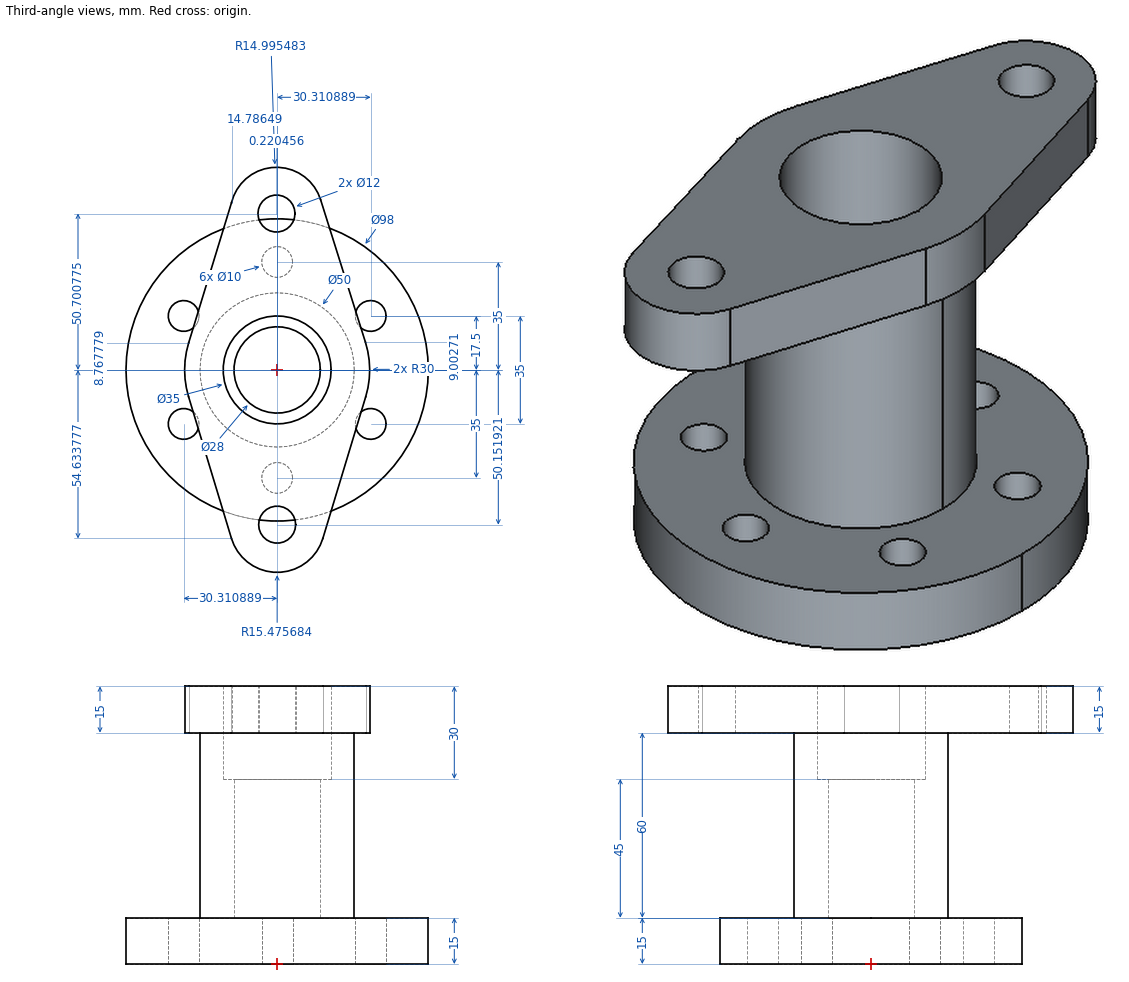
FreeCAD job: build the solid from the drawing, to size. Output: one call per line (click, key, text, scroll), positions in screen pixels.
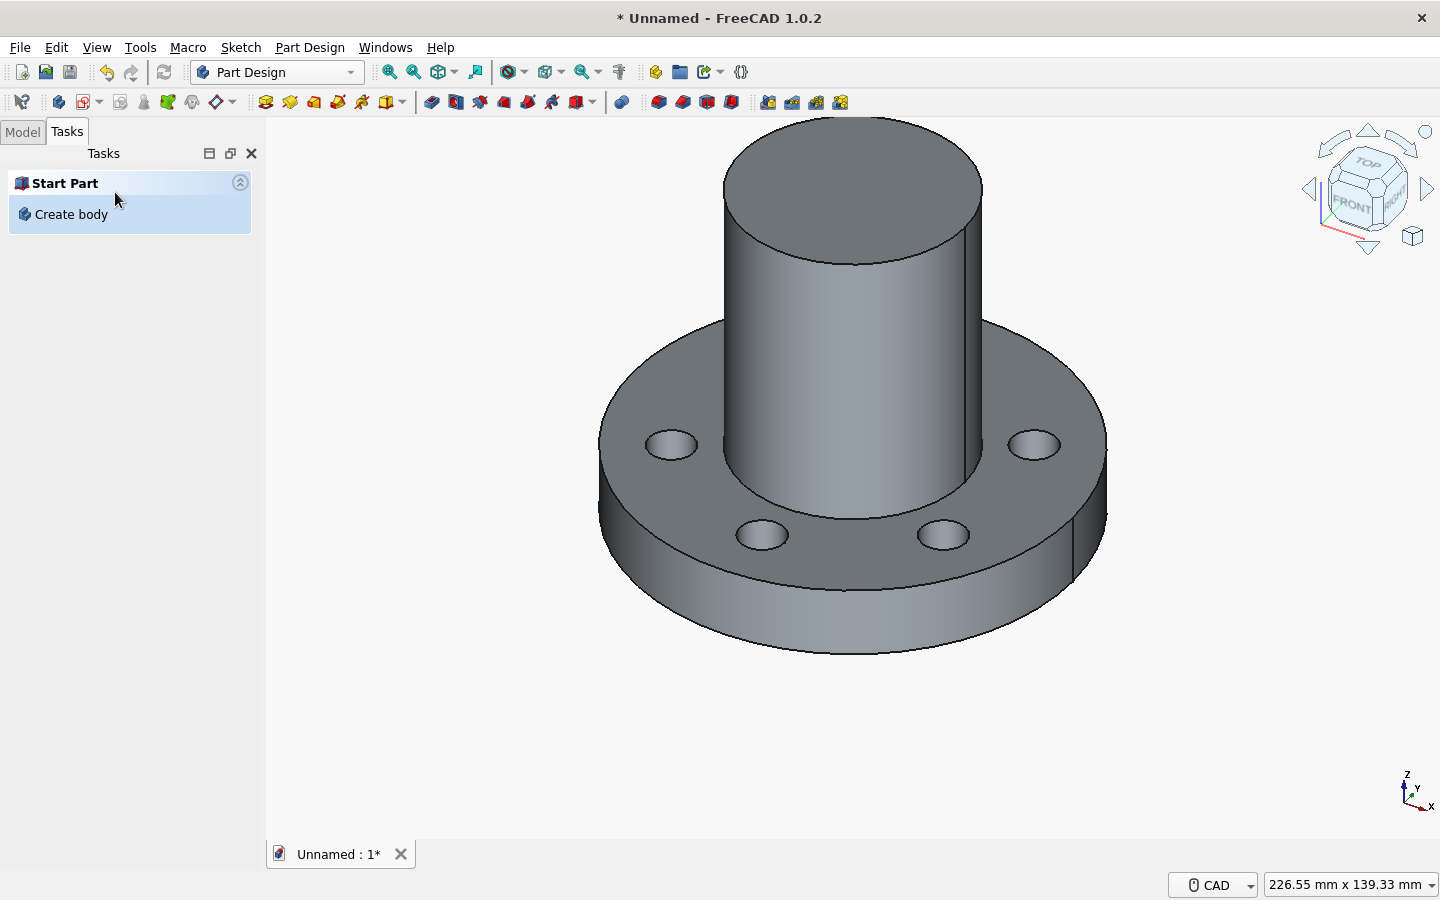
click(390, 72)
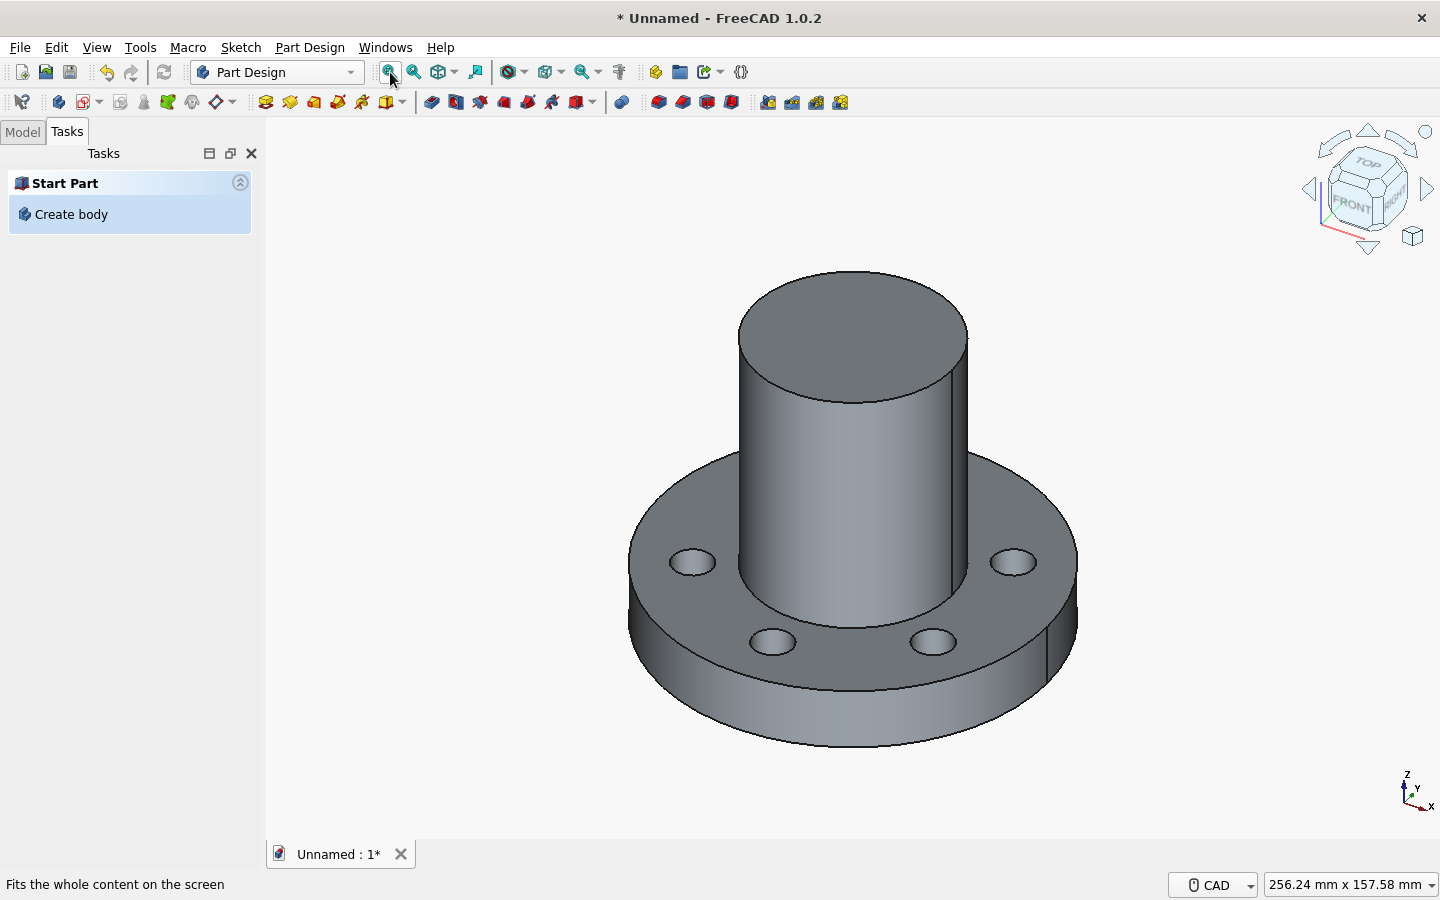
click(853, 336)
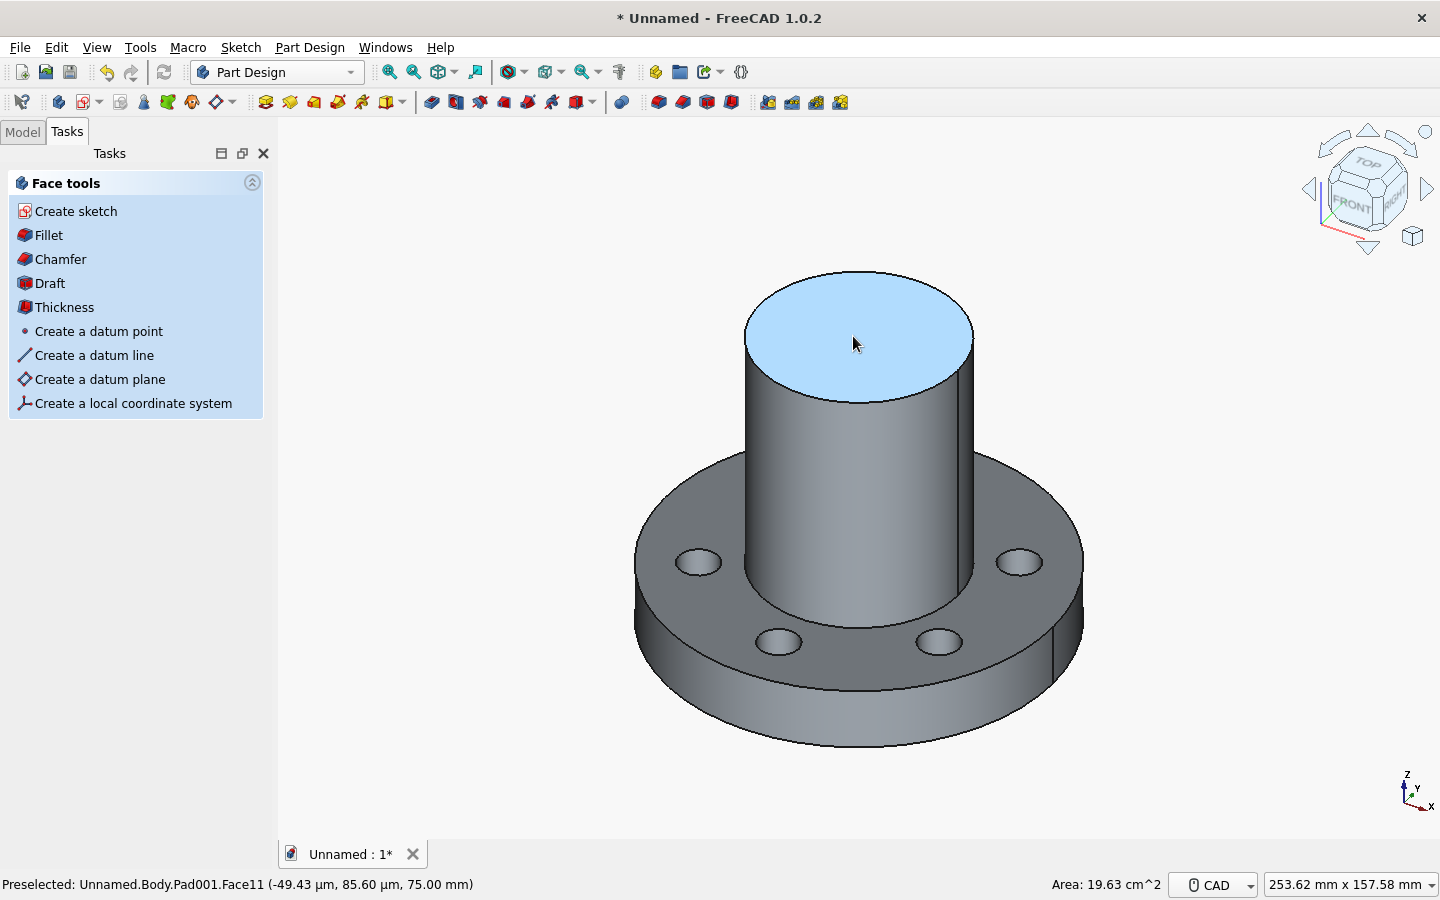
click(84, 102)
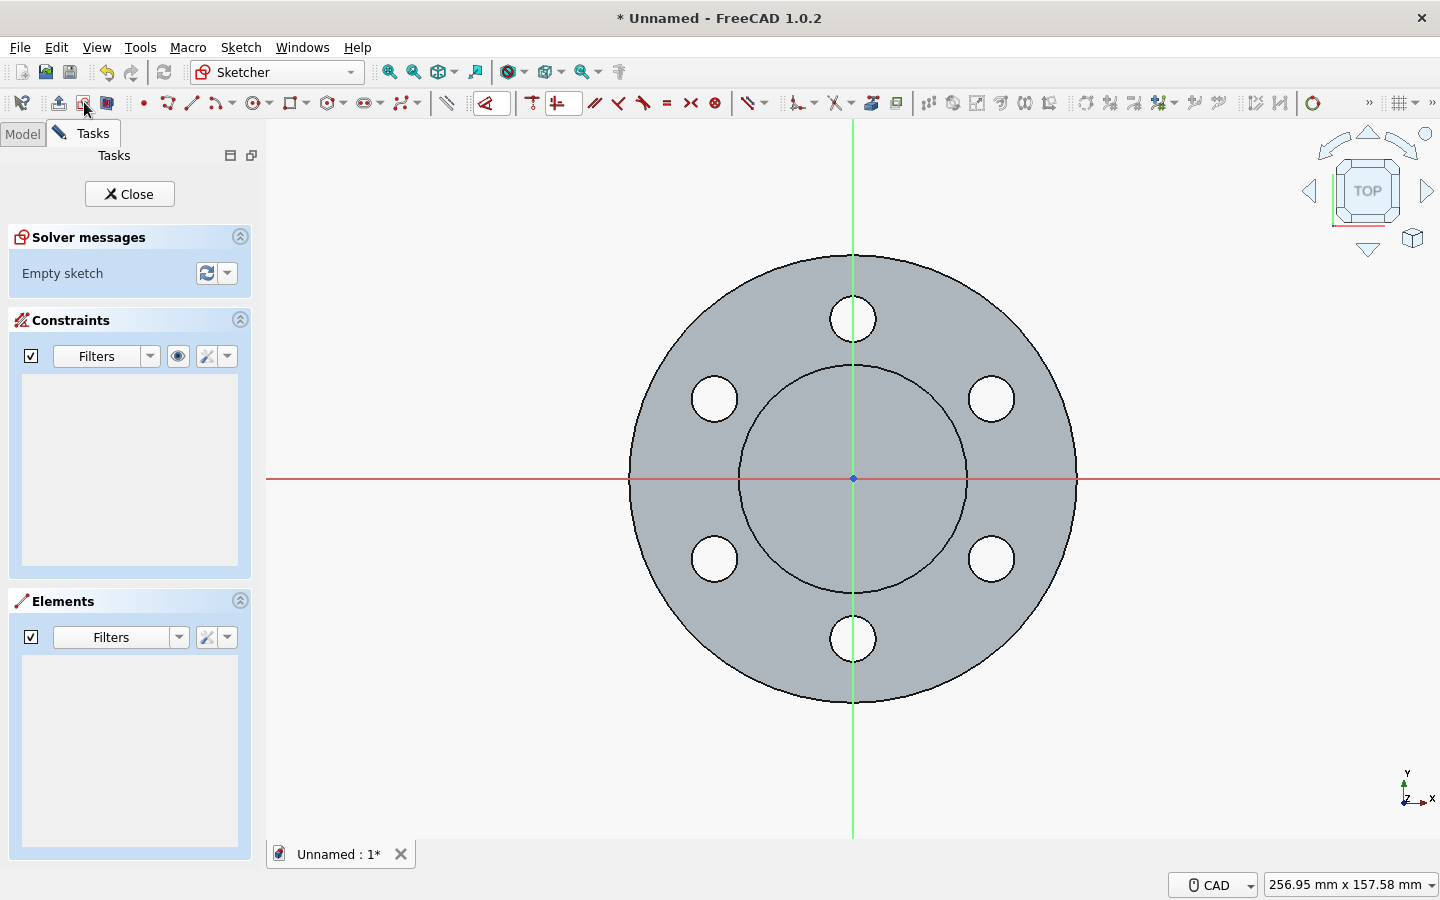
click(192, 104)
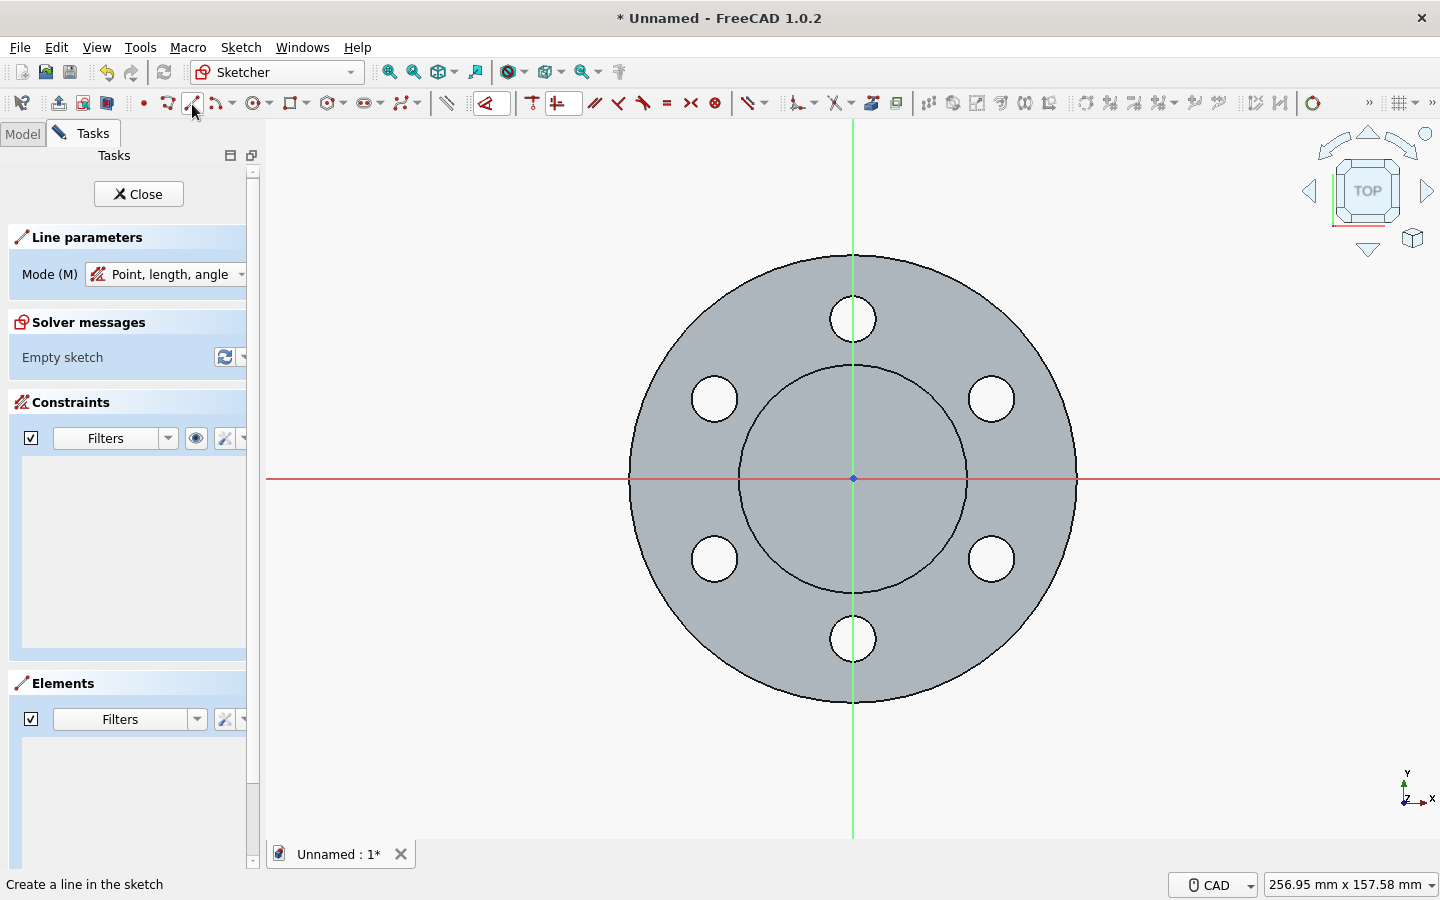
click(722, 519)
click(785, 729)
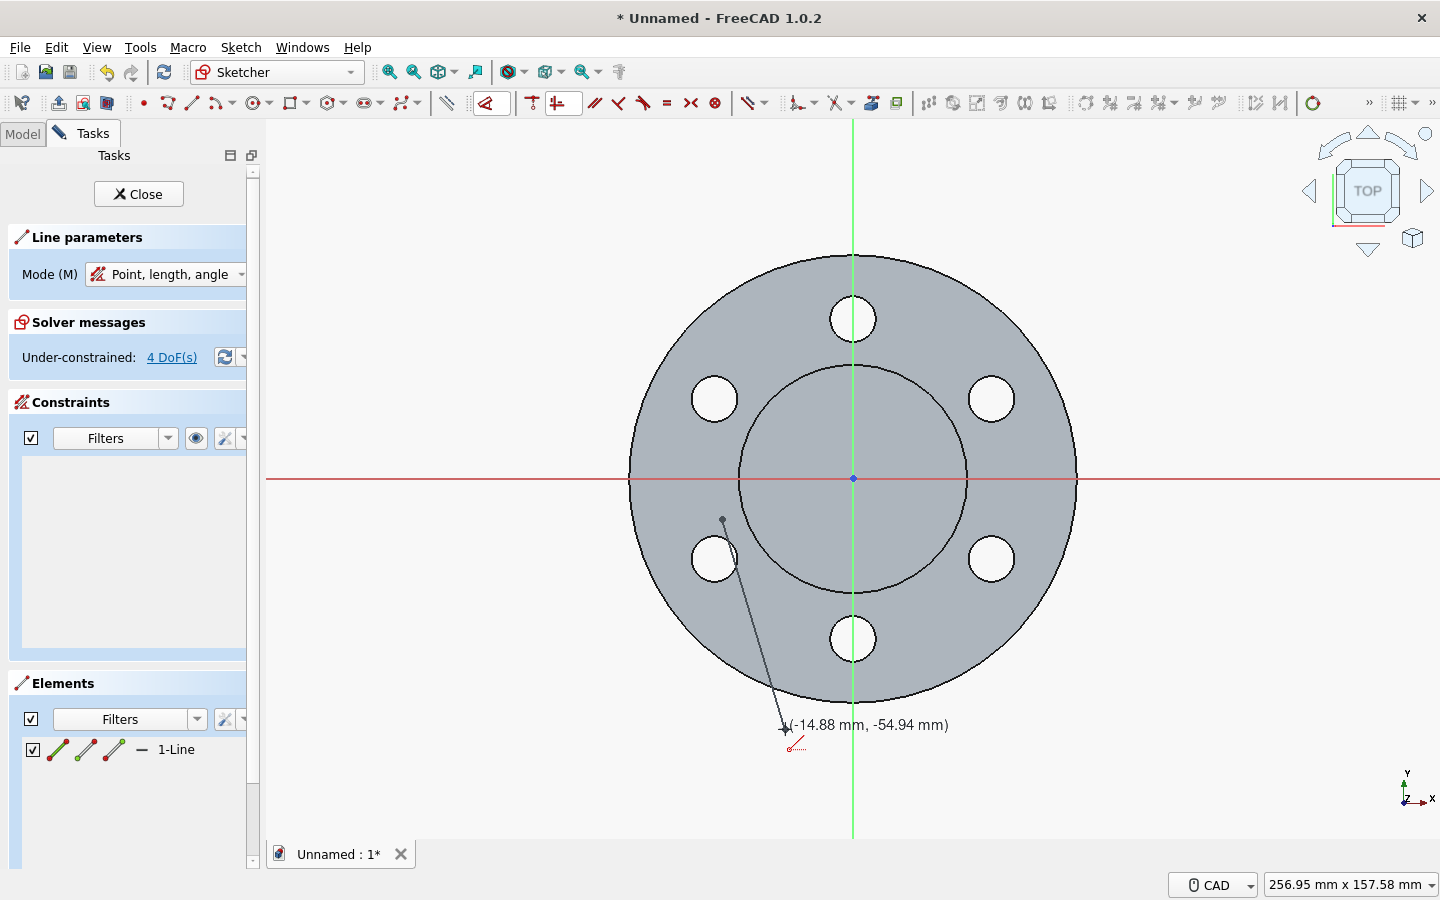
click(921, 729)
click(984, 519)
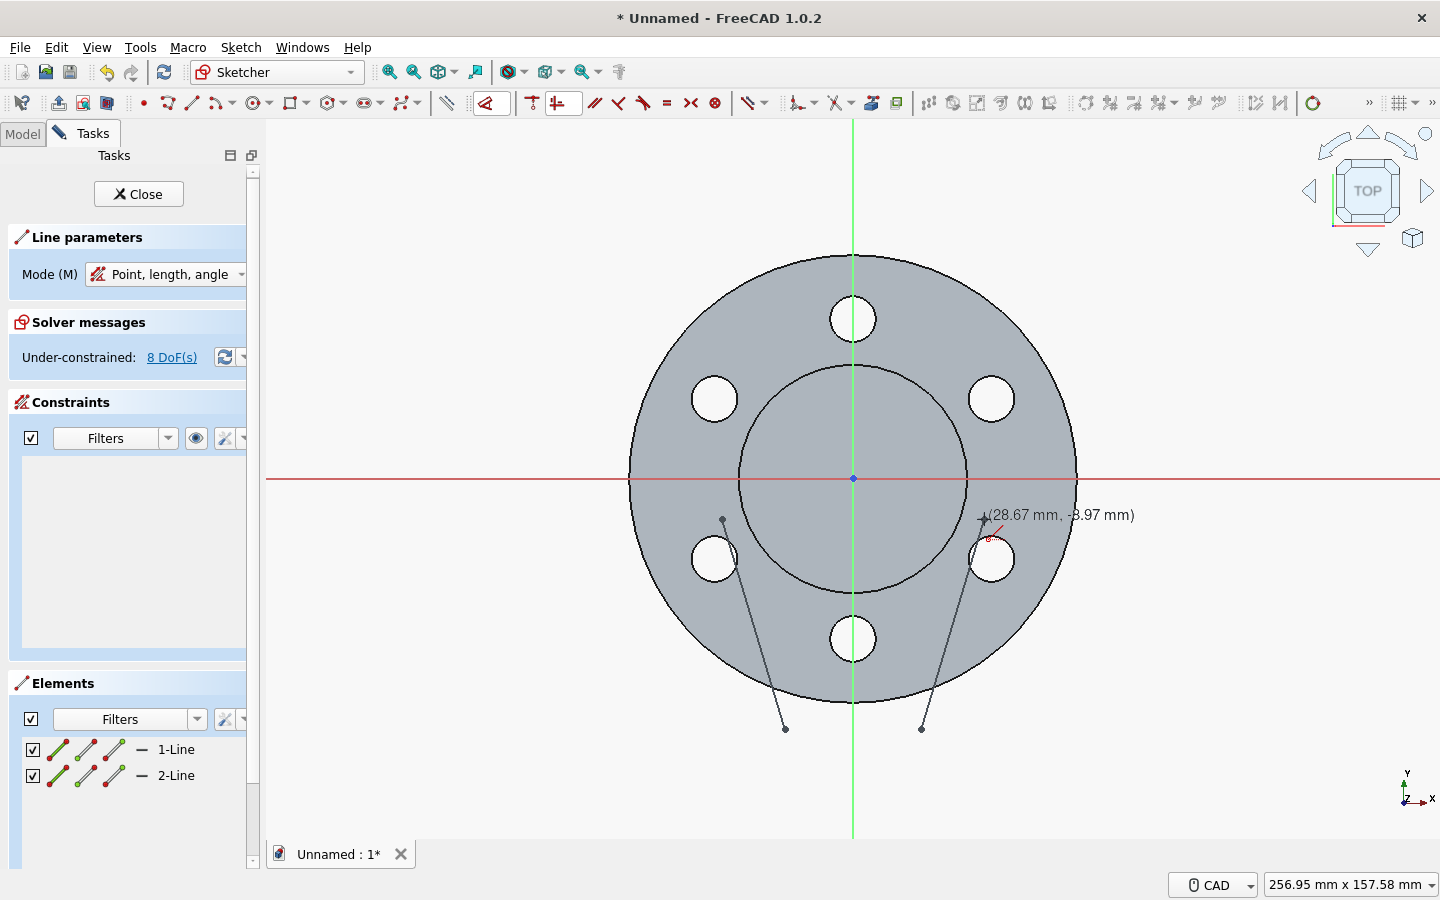
click(984, 438)
click(917, 227)